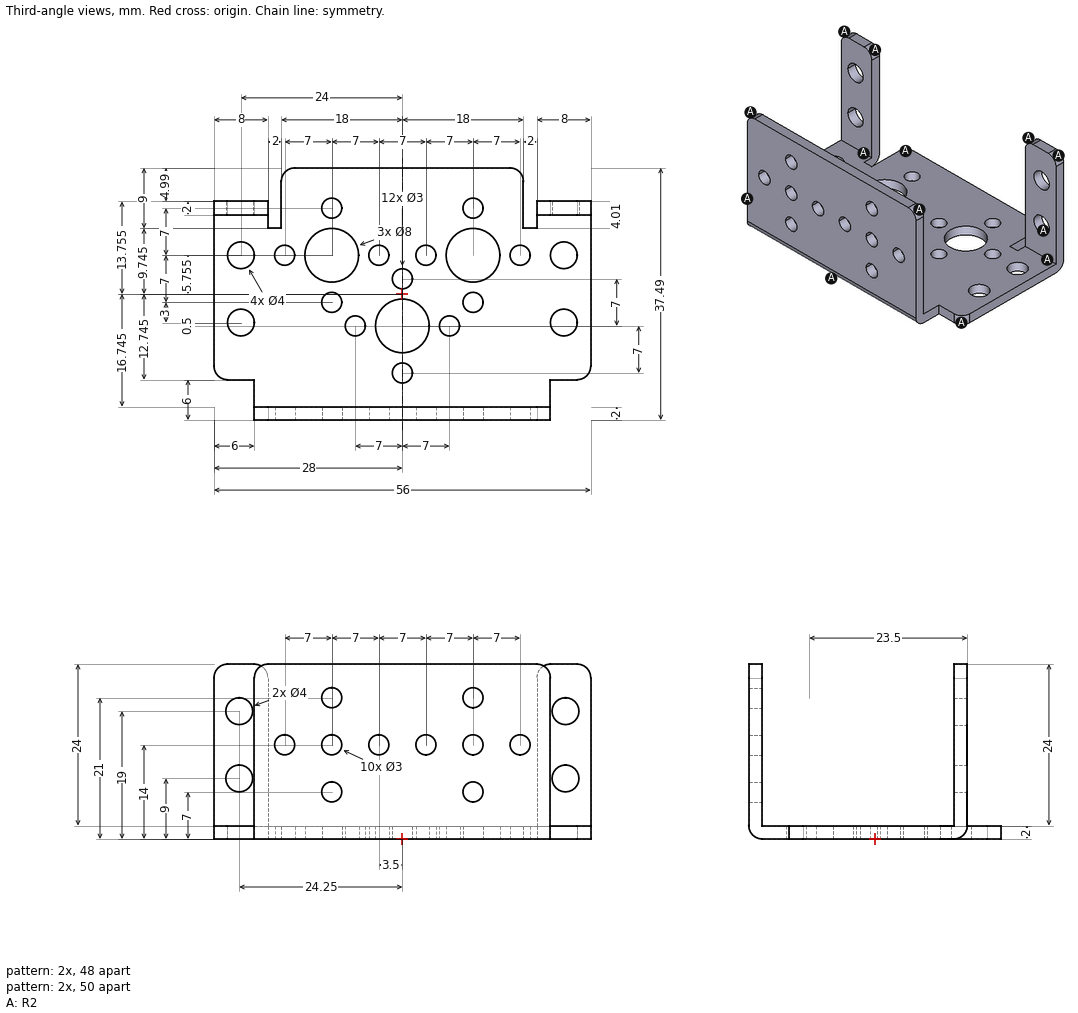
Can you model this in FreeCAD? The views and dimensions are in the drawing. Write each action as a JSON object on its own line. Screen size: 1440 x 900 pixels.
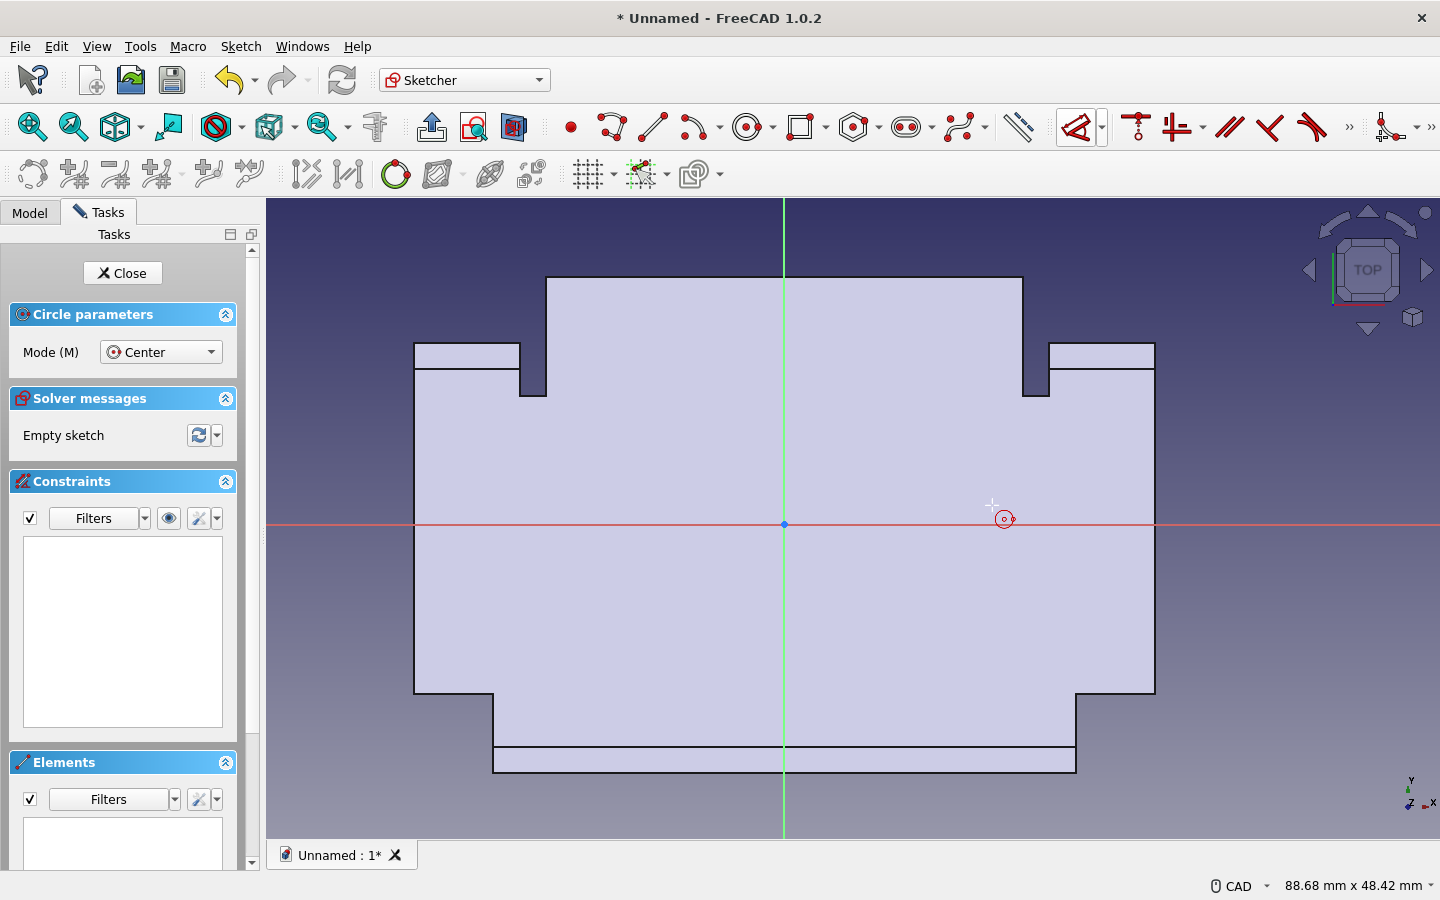
{"action": "left_click", "coordinate": [467, 449]}
{"action": "mouse_move", "coordinate": [485, 430]}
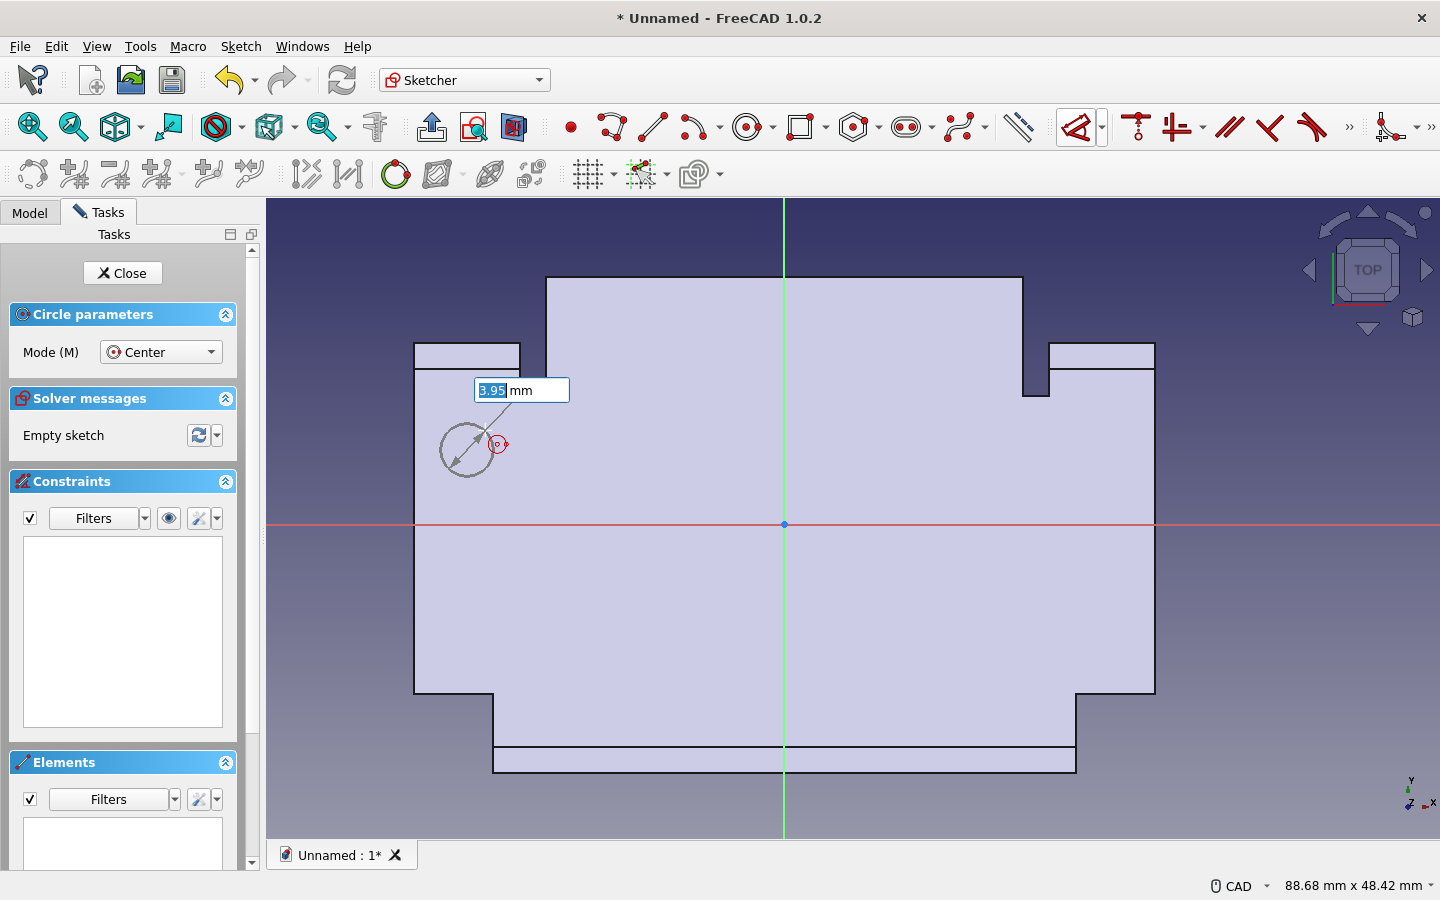
{"action": "type", "text": "4"}
{"action": "key", "text": "Return"}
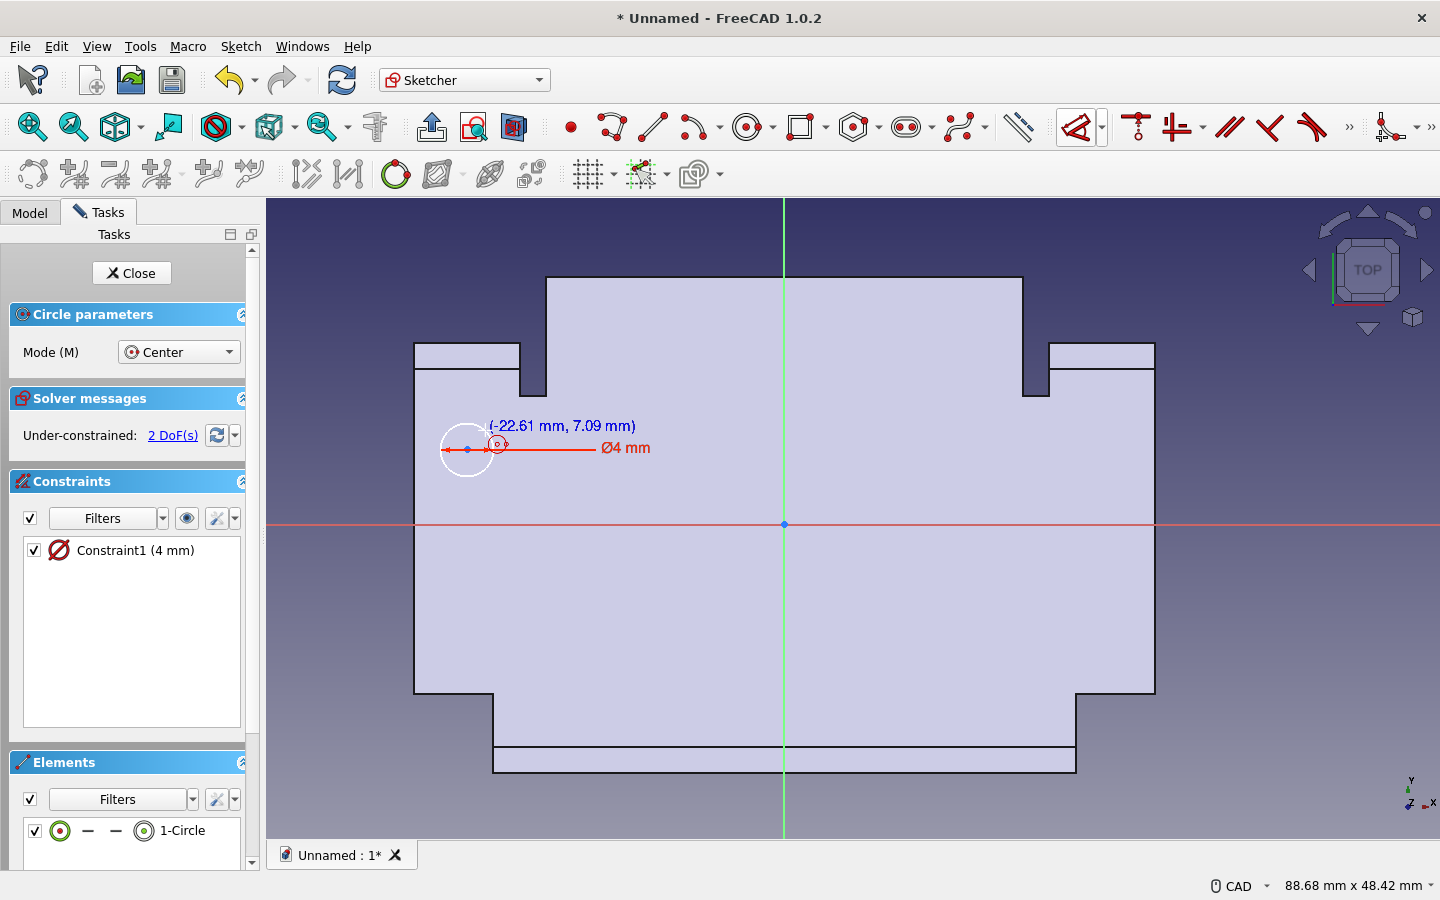
{"action": "left_click", "coordinate": [467, 581]}
{"action": "mouse_move", "coordinate": [485, 562]}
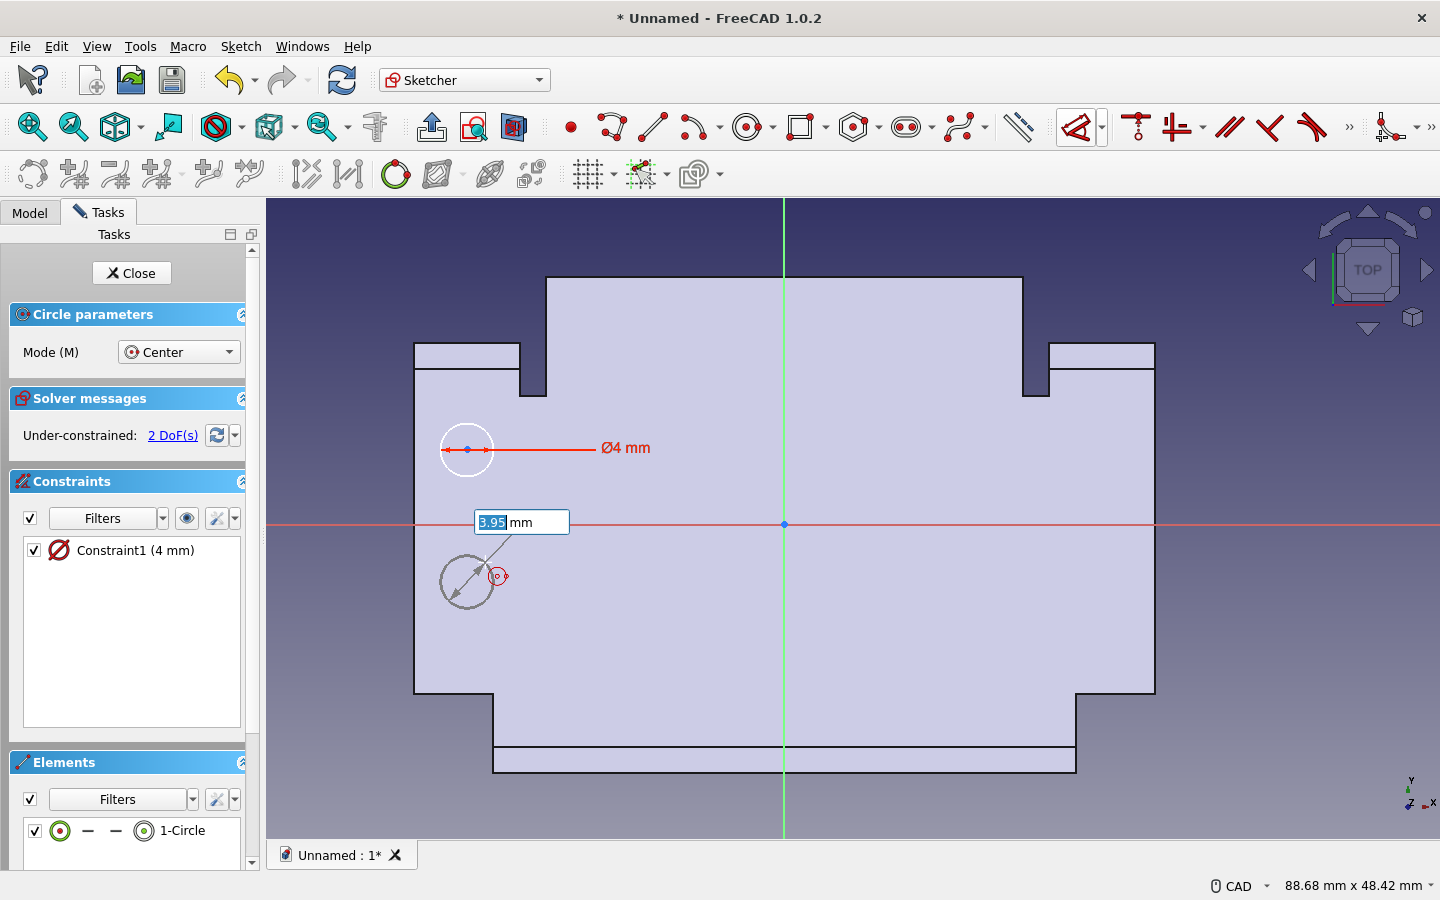
{"action": "type", "text": "4"}
{"action": "key", "text": "Return"}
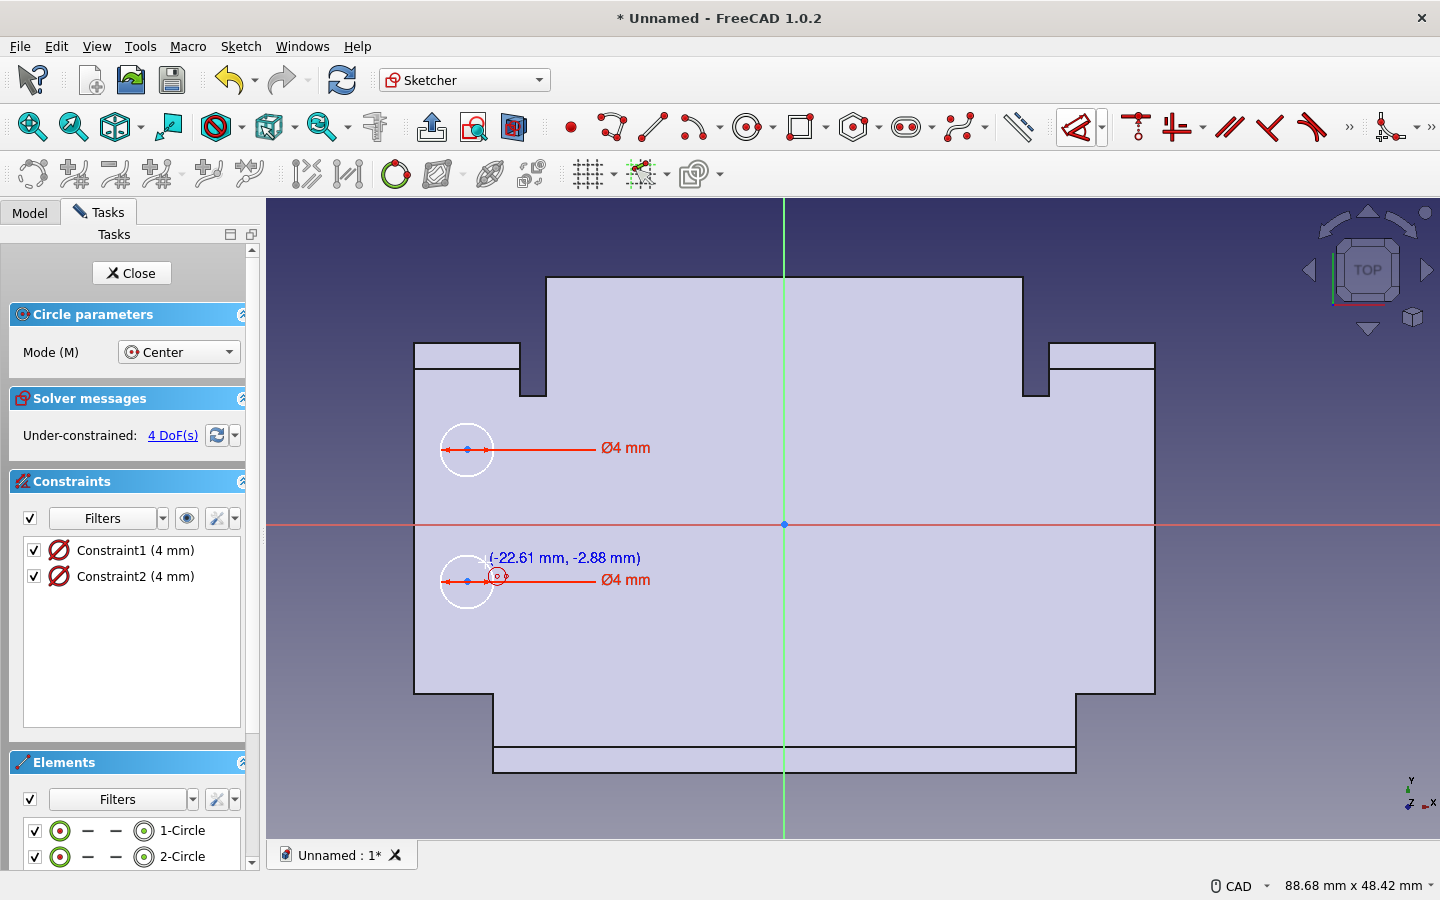
{"action": "left_click", "coordinate": [645, 449]}
{"action": "mouse_move", "coordinate": [683, 411]}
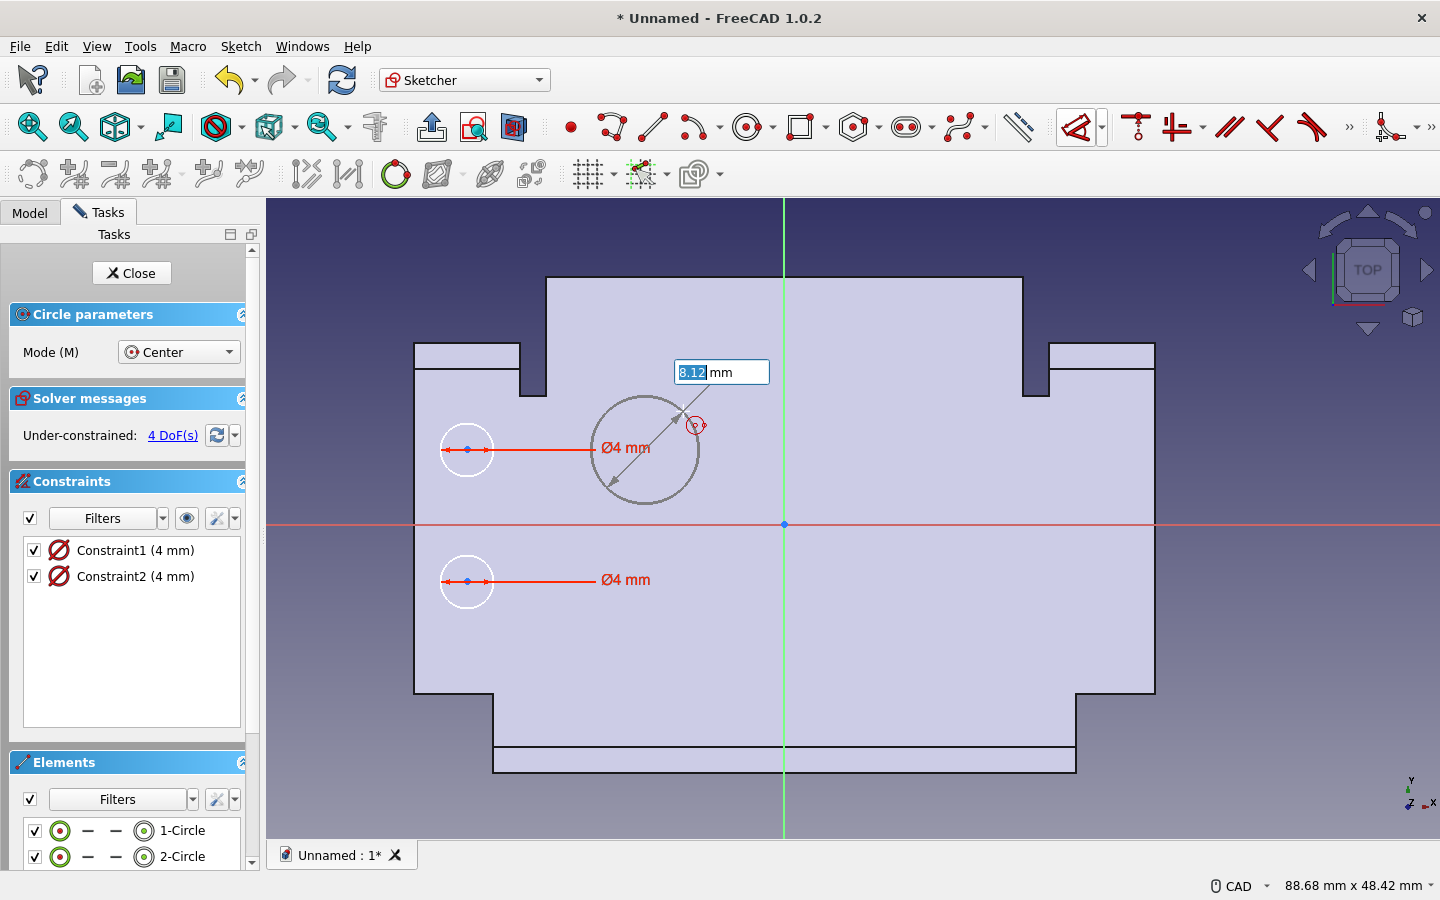
{"action": "type", "text": "8"}
{"action": "key", "text": "Return"}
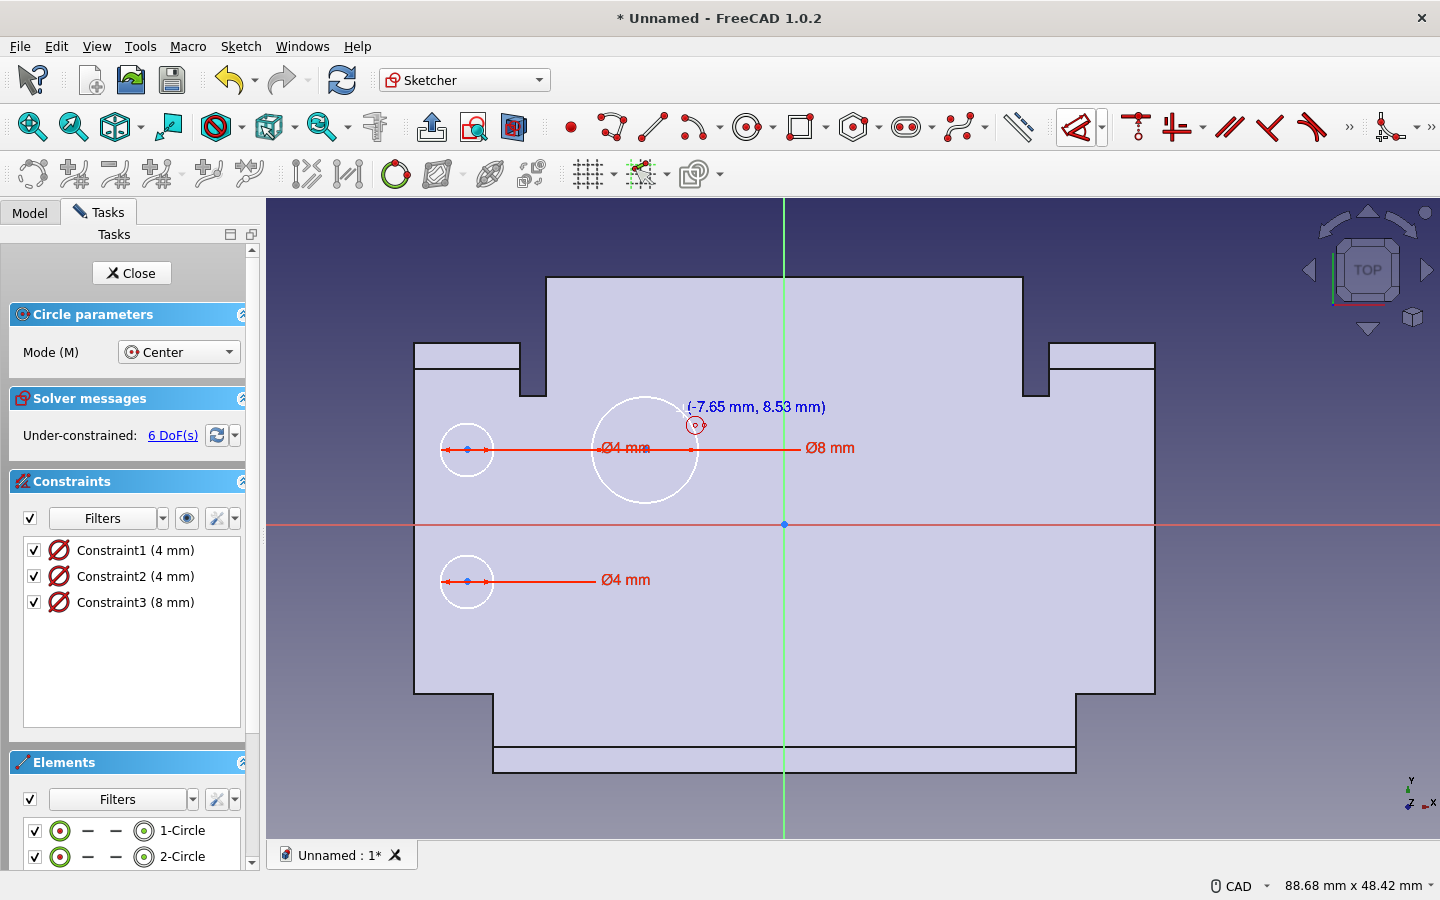
{"action": "left_click", "coordinate": [784, 588]}
{"action": "mouse_move", "coordinate": [822, 550]}